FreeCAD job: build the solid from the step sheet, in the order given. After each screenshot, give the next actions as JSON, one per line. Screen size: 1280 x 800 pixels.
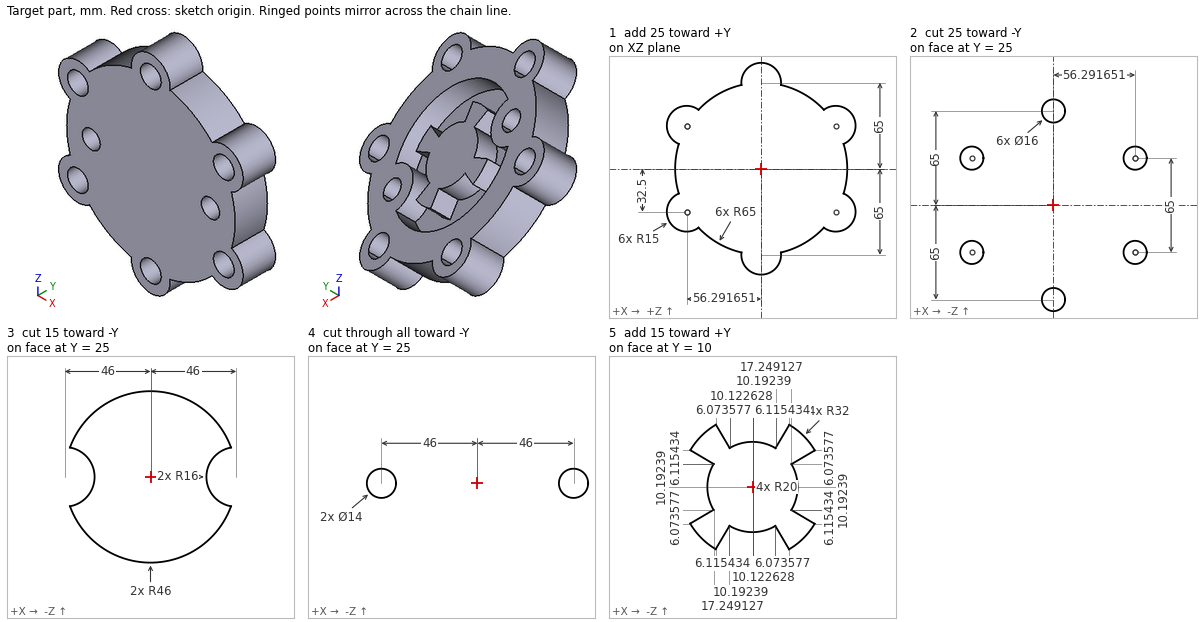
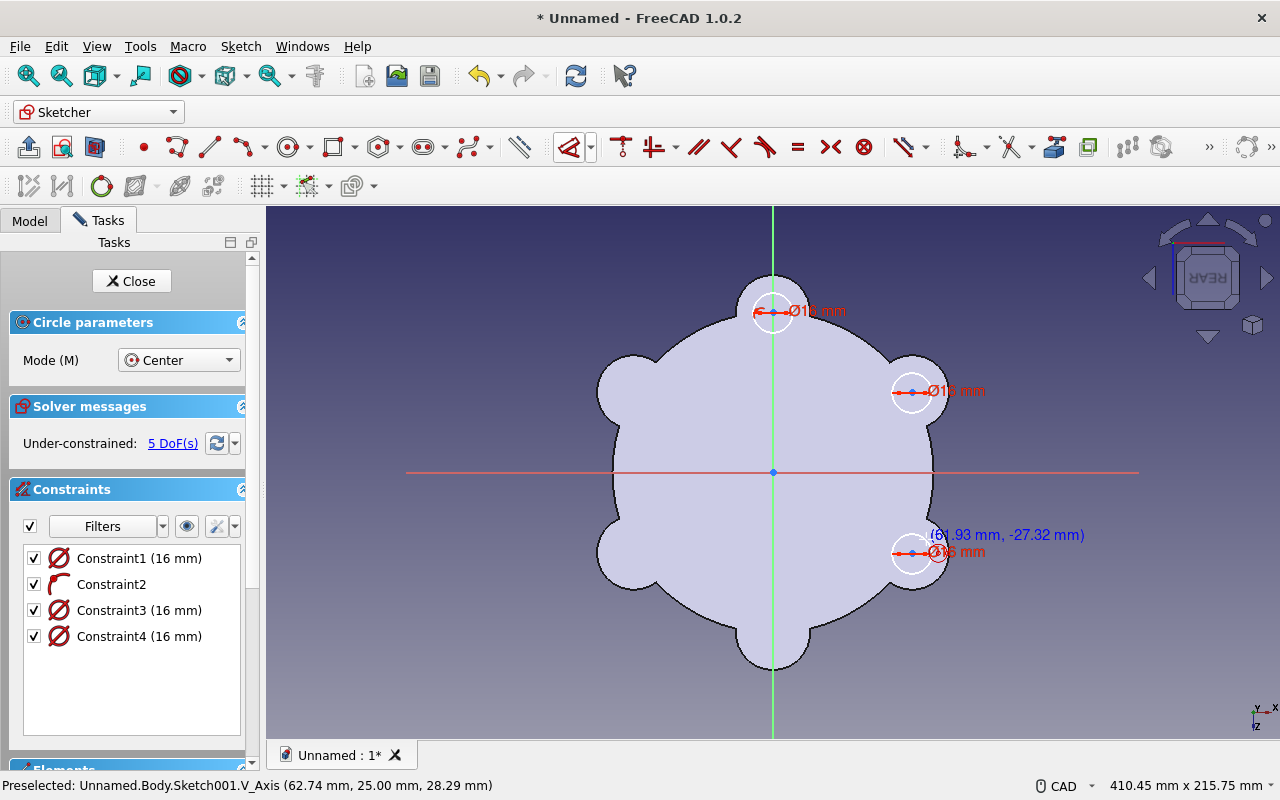
{"action": "left_click", "coordinate": [773, 633]}
{"action": "mouse_move", "coordinate": [792, 626]}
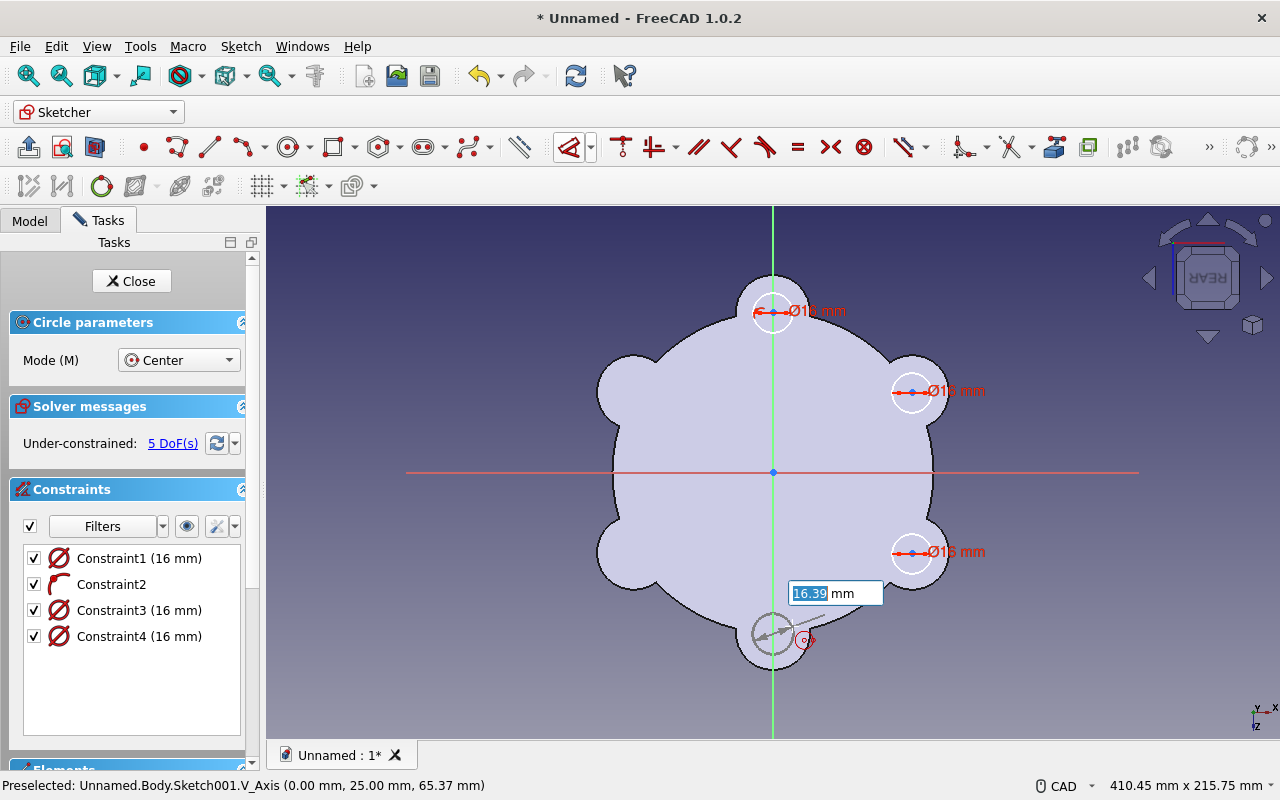
{"action": "type", "text": "16"}
{"action": "key", "text": "Return"}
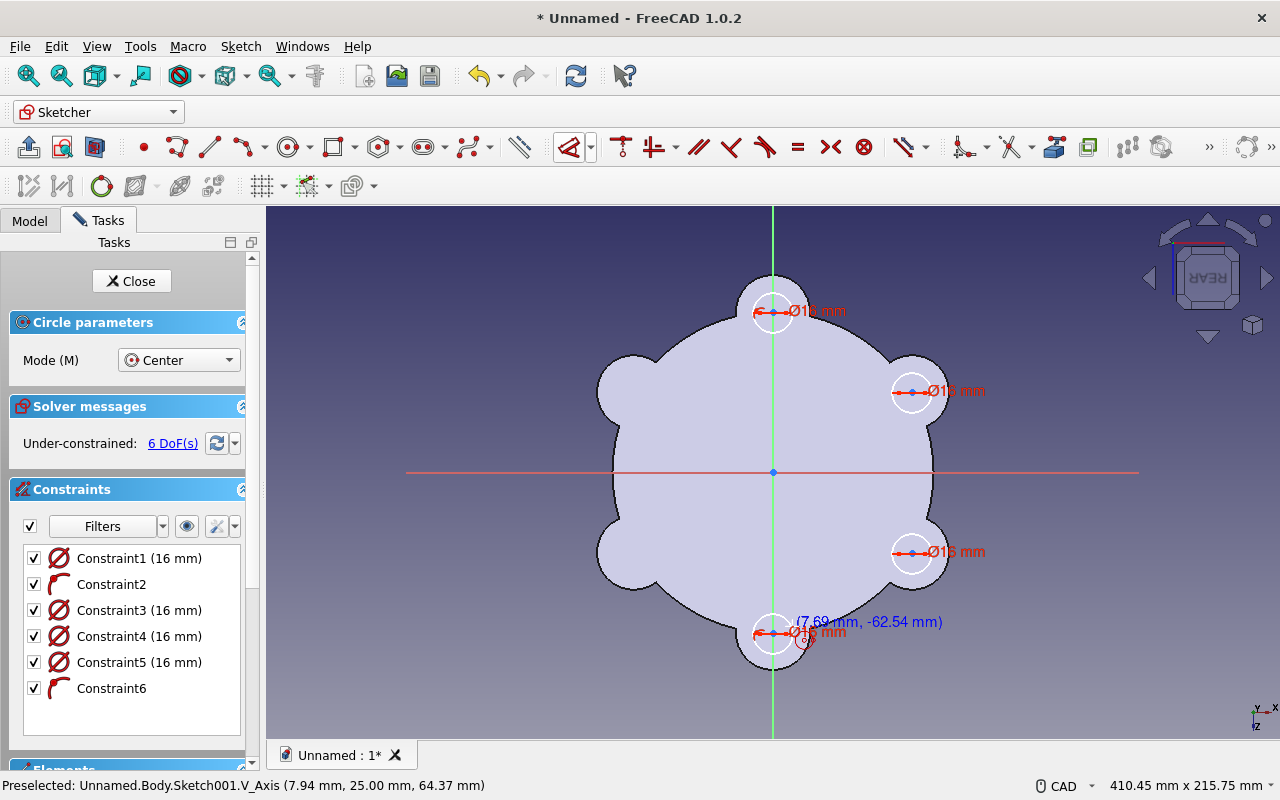
{"action": "left_click", "coordinate": [634, 553]}
{"action": "mouse_move", "coordinate": [648, 539]}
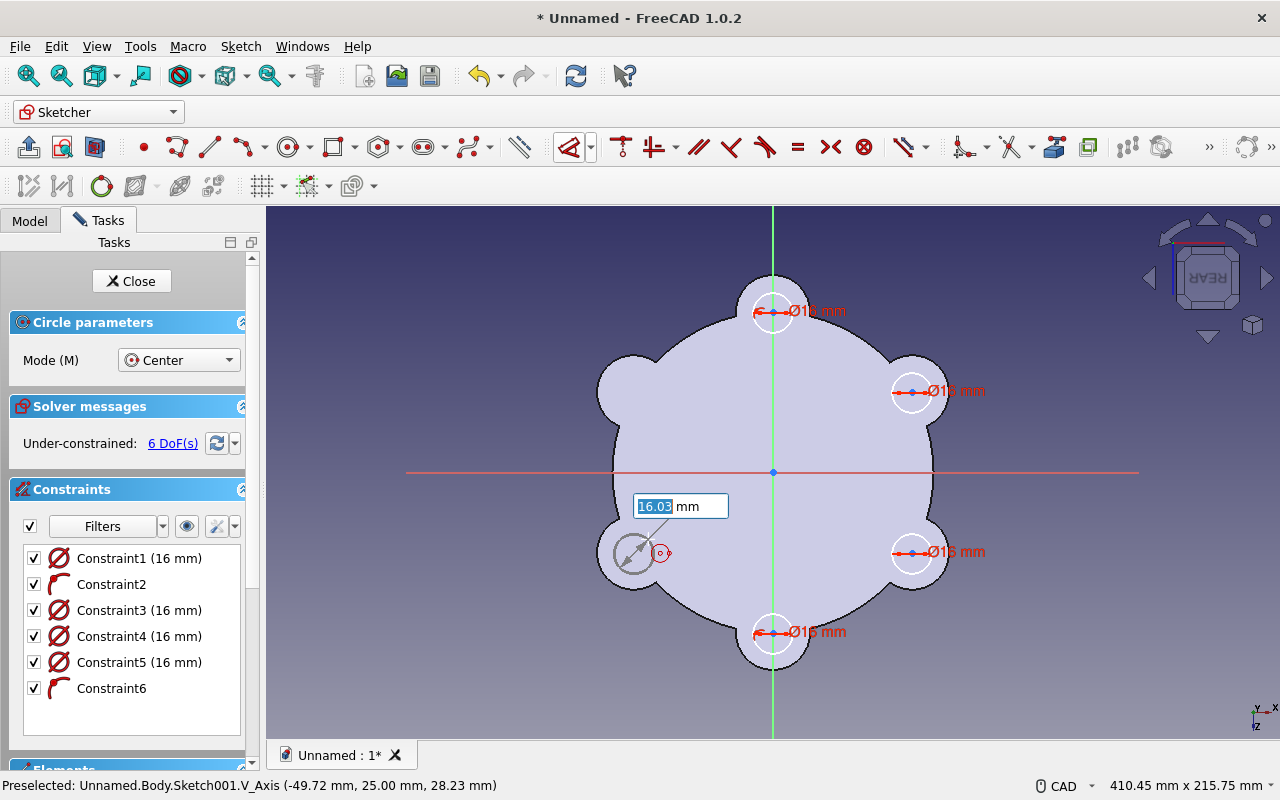
{"action": "type", "text": "16"}
{"action": "key", "text": "Return"}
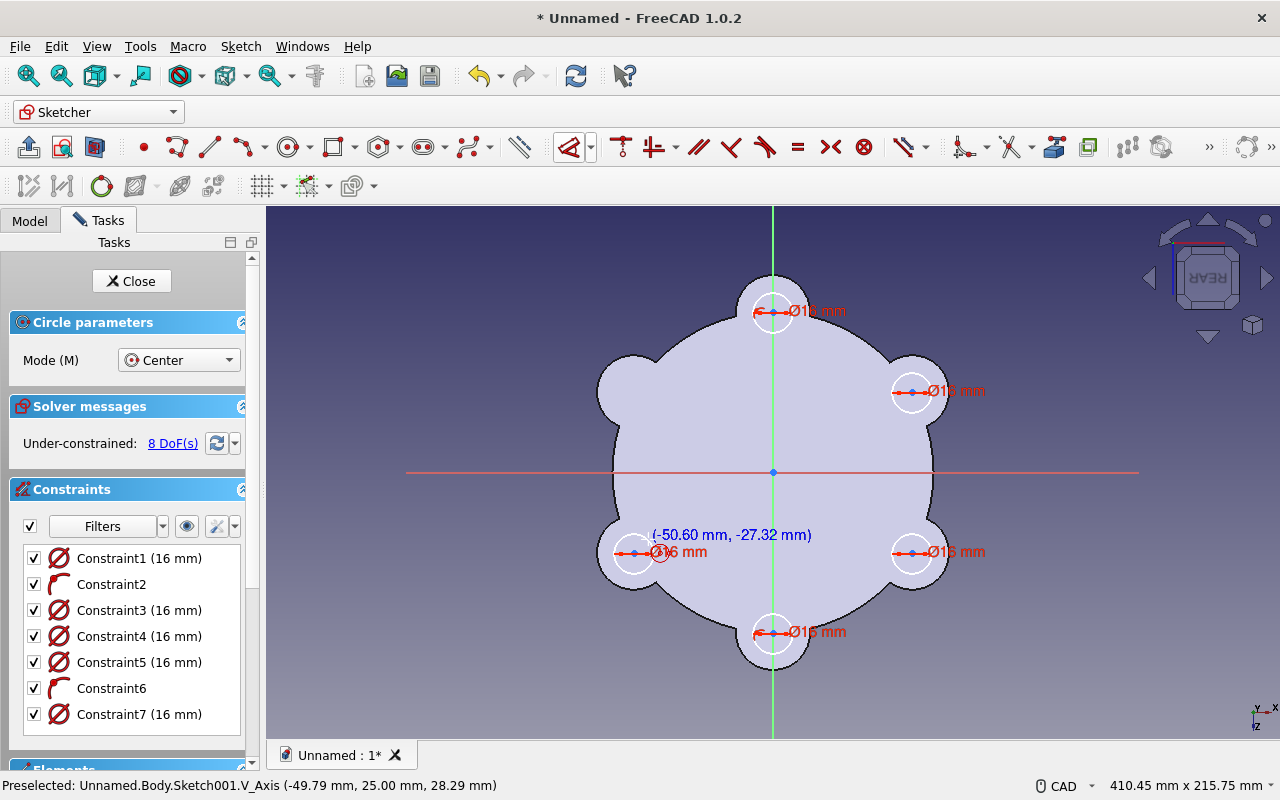
{"action": "left_click", "coordinate": [634, 392]}
{"action": "mouse_move", "coordinate": [648, 378]}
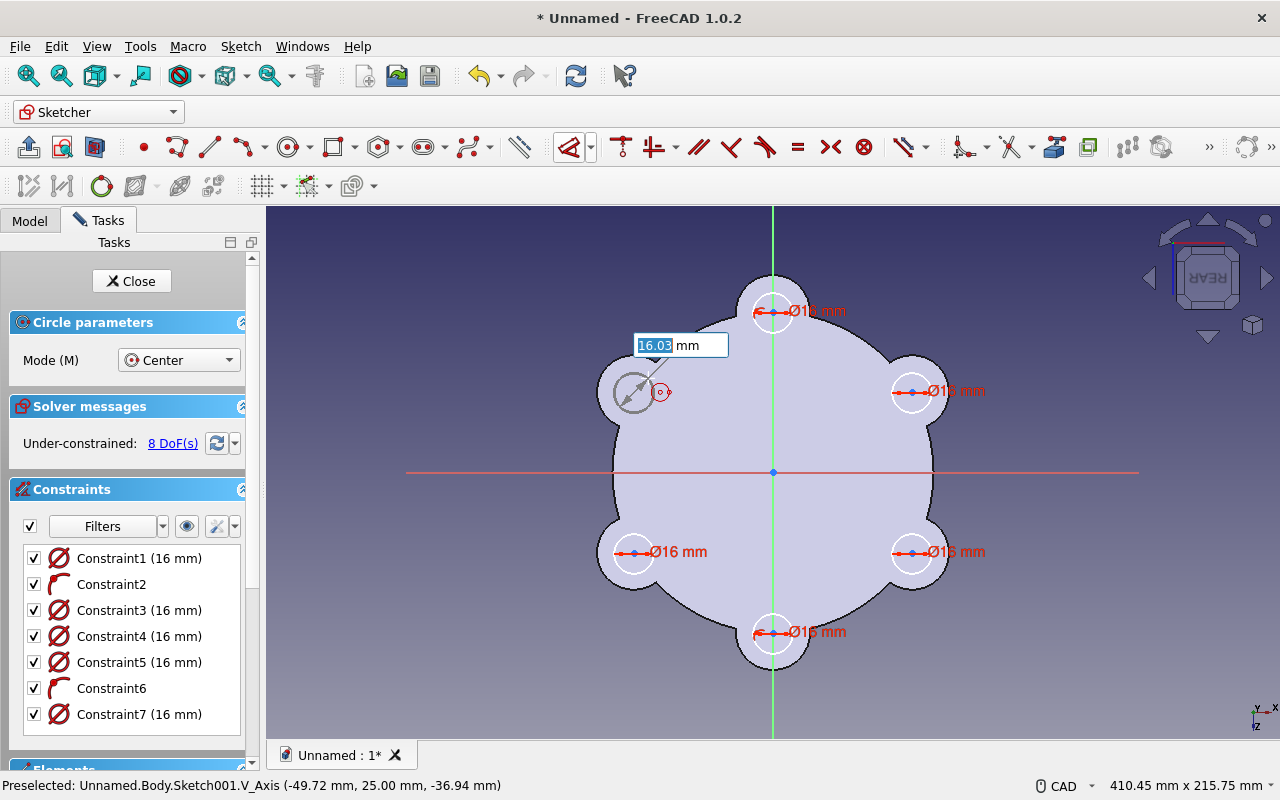
{"action": "type", "text": "16"}
{"action": "key", "text": "Return"}
{"action": "key", "text": "Escape"}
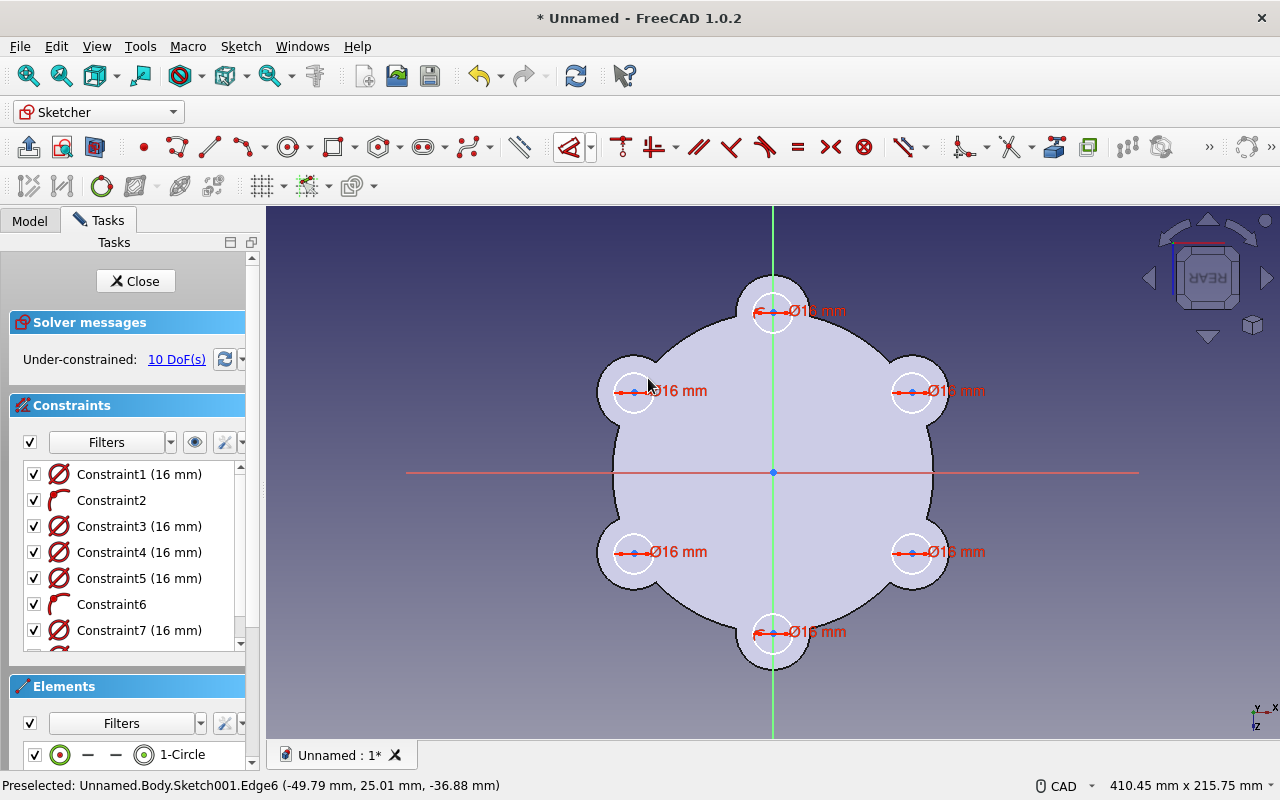
{"action": "left_click", "coordinate": [912, 393]}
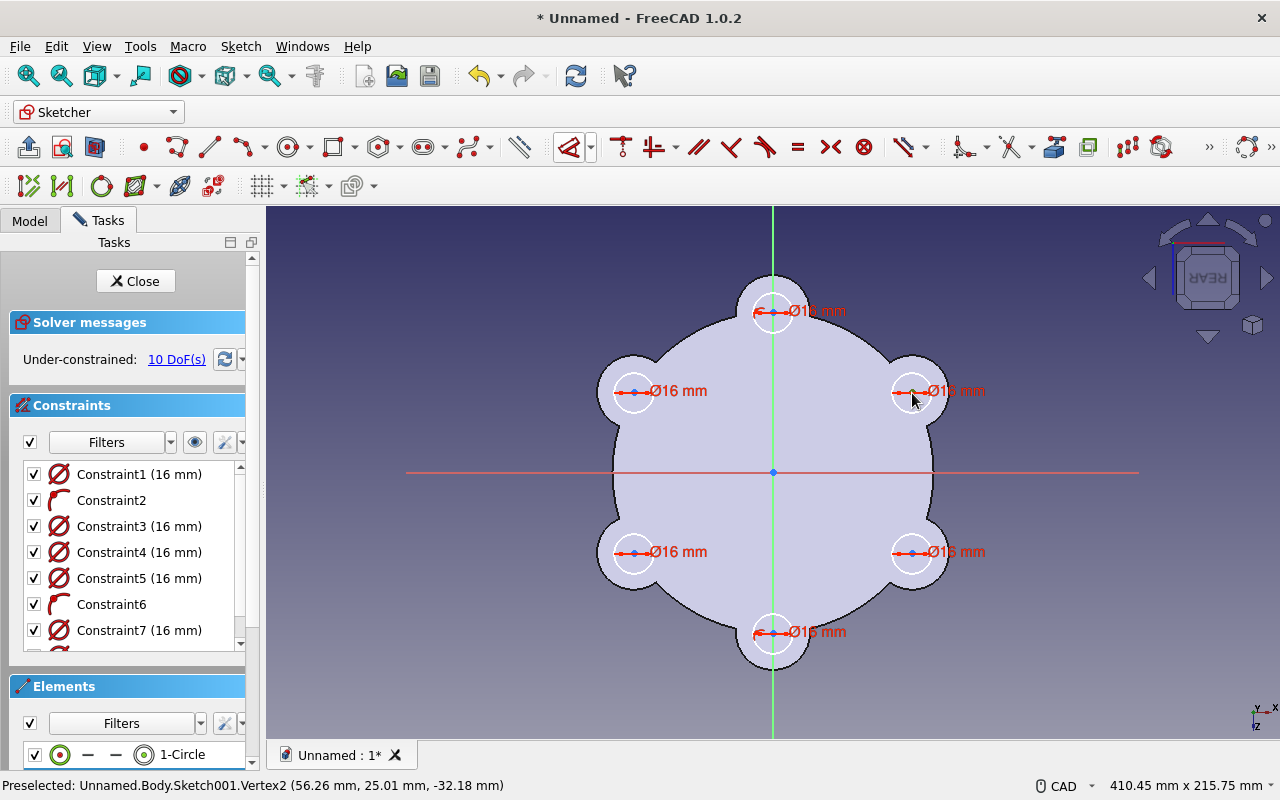
{"action": "left_click", "coordinate": [912, 554]}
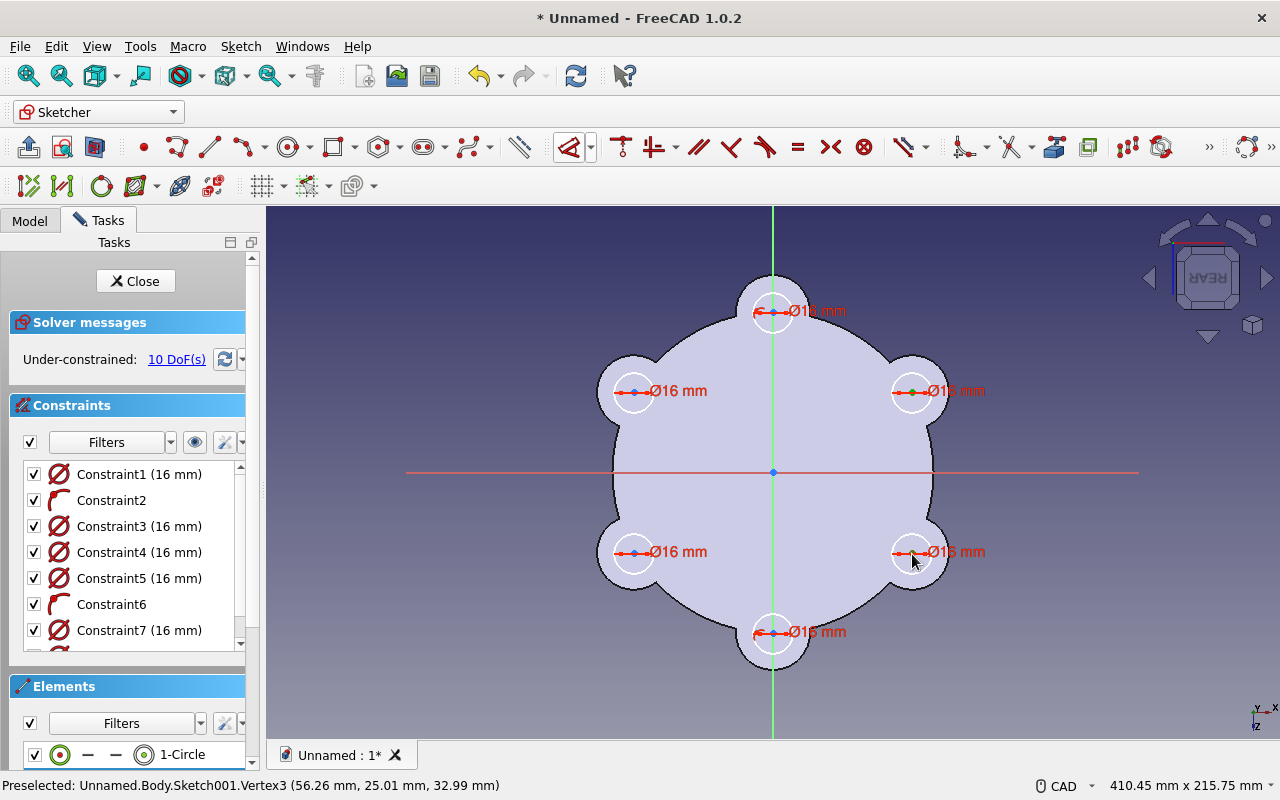
{"action": "left_click", "coordinate": [411, 473]}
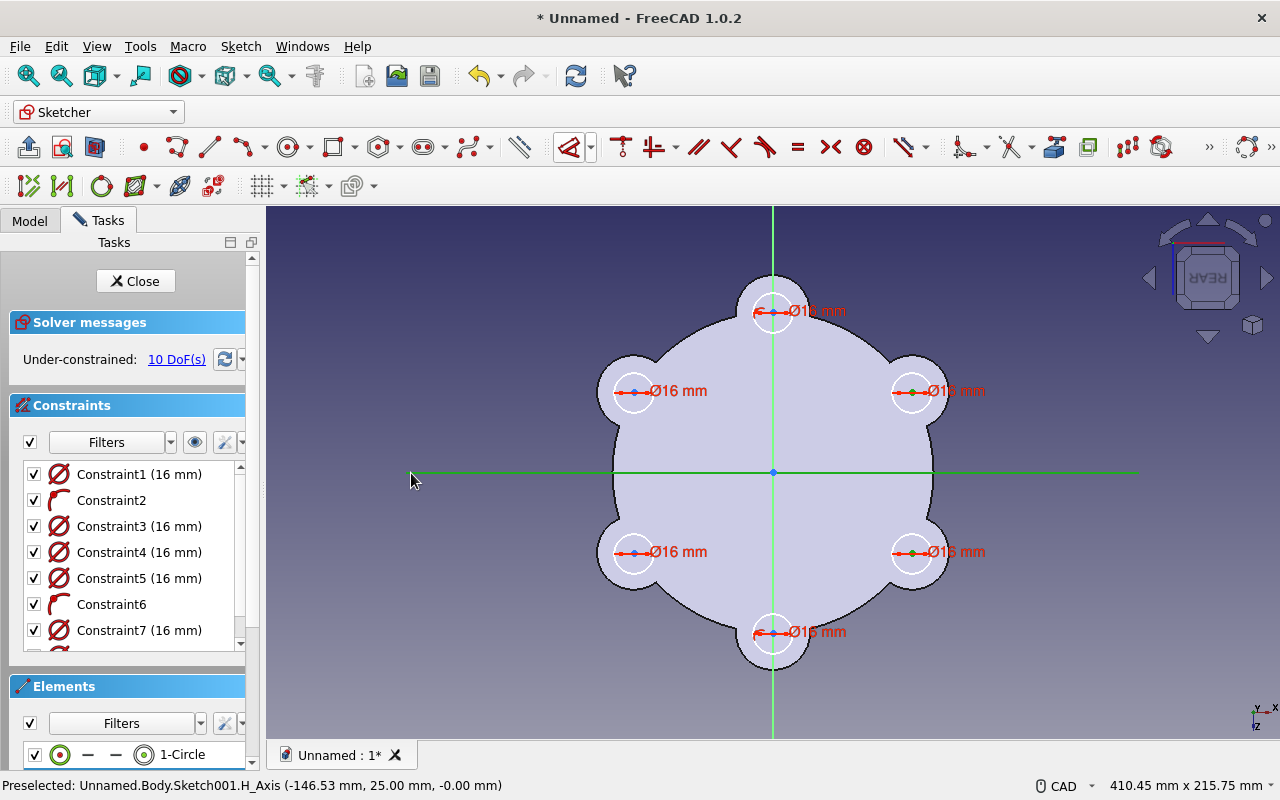
{"action": "left_click", "coordinate": [831, 148]}